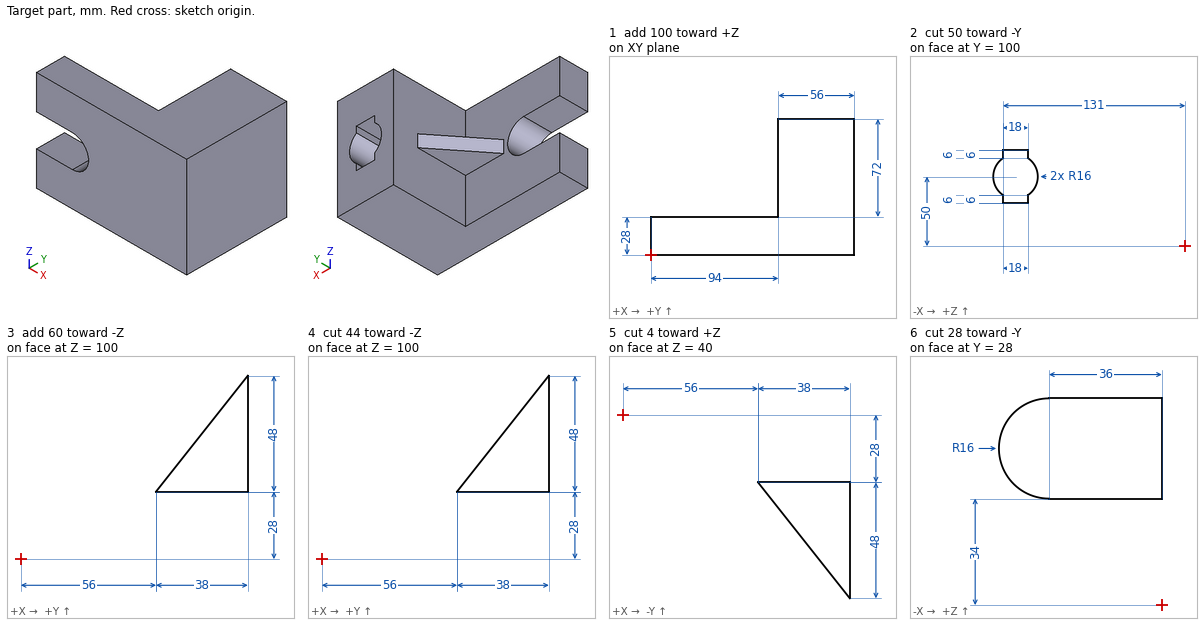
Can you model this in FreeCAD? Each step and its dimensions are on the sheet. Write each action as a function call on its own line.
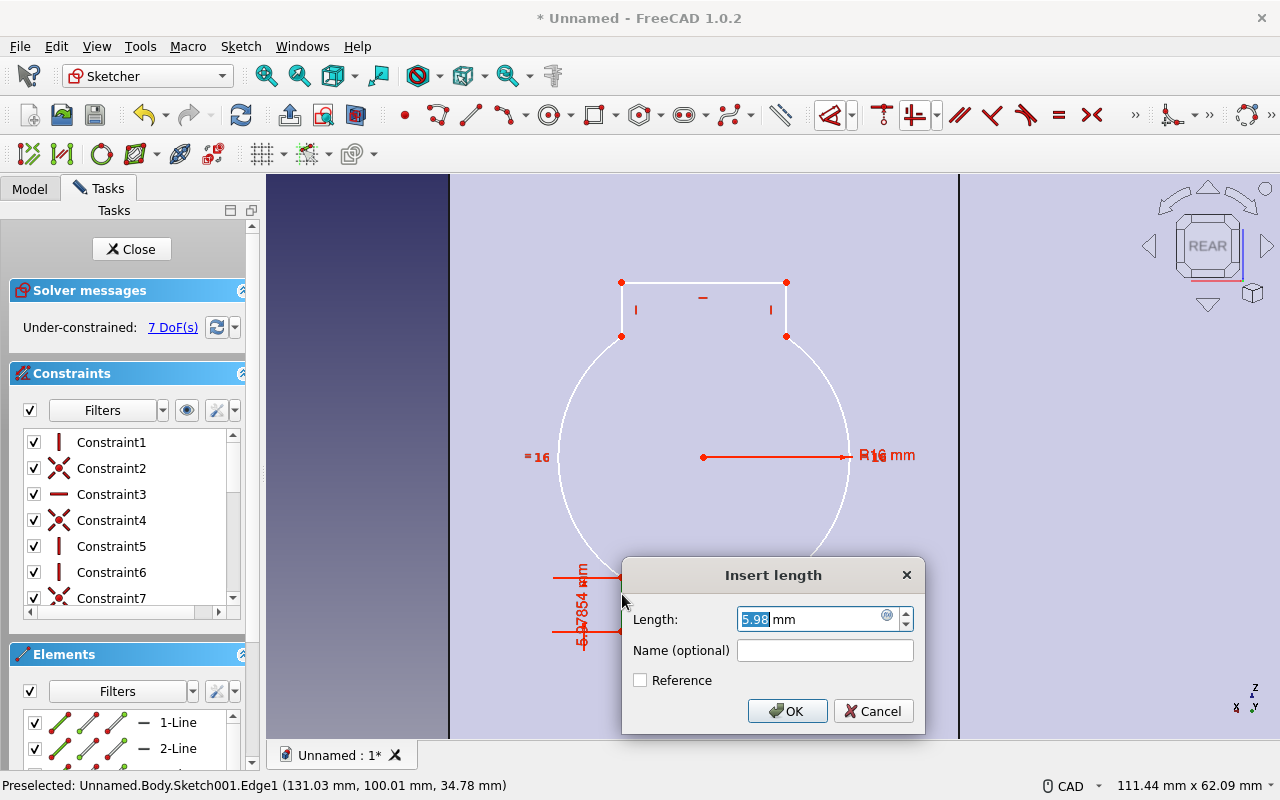
text(6)
key(Return)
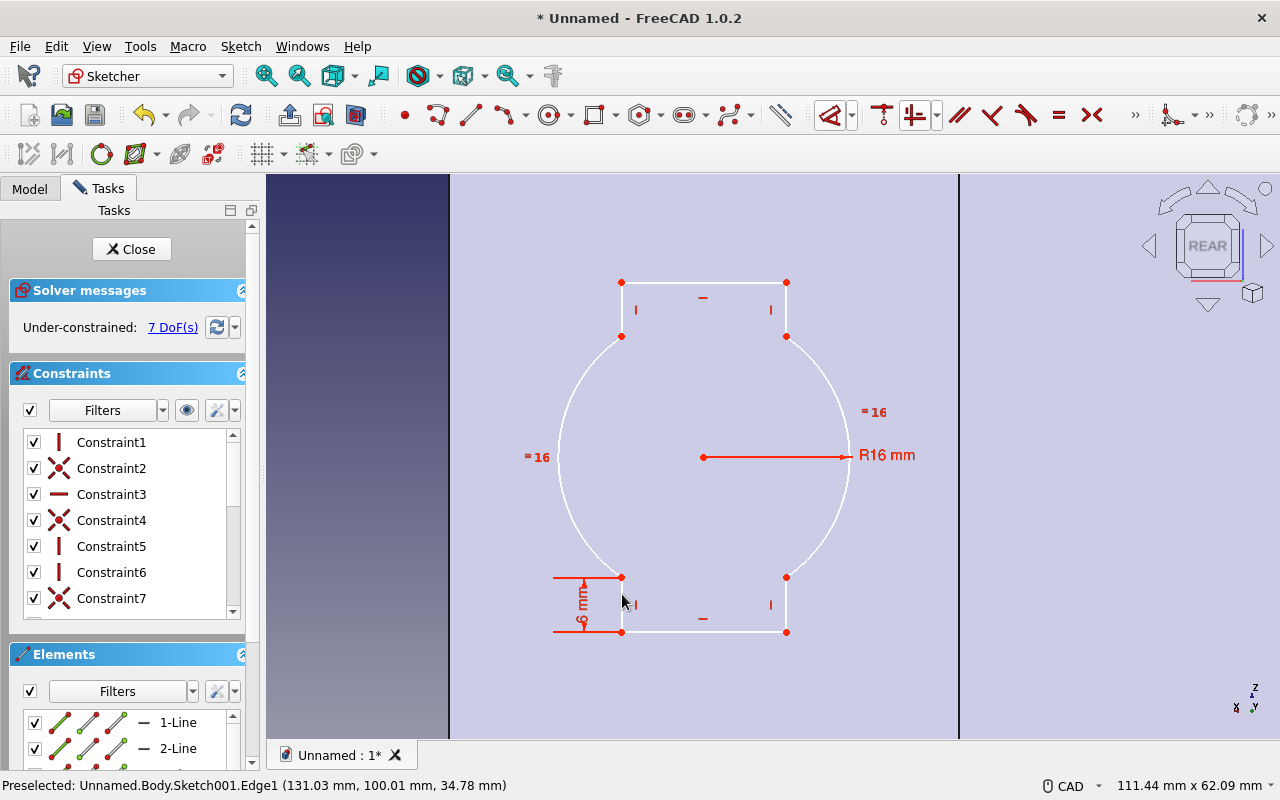
click(786, 616)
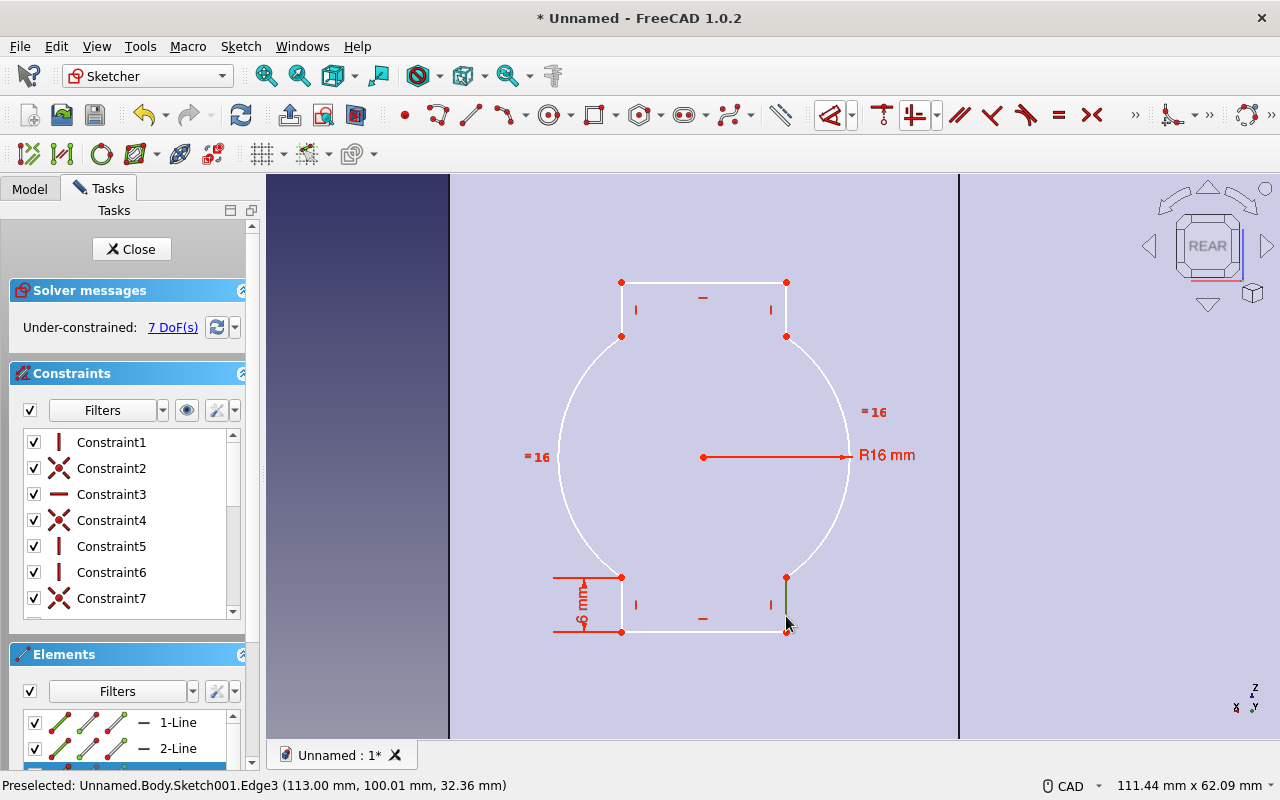
click(852, 116)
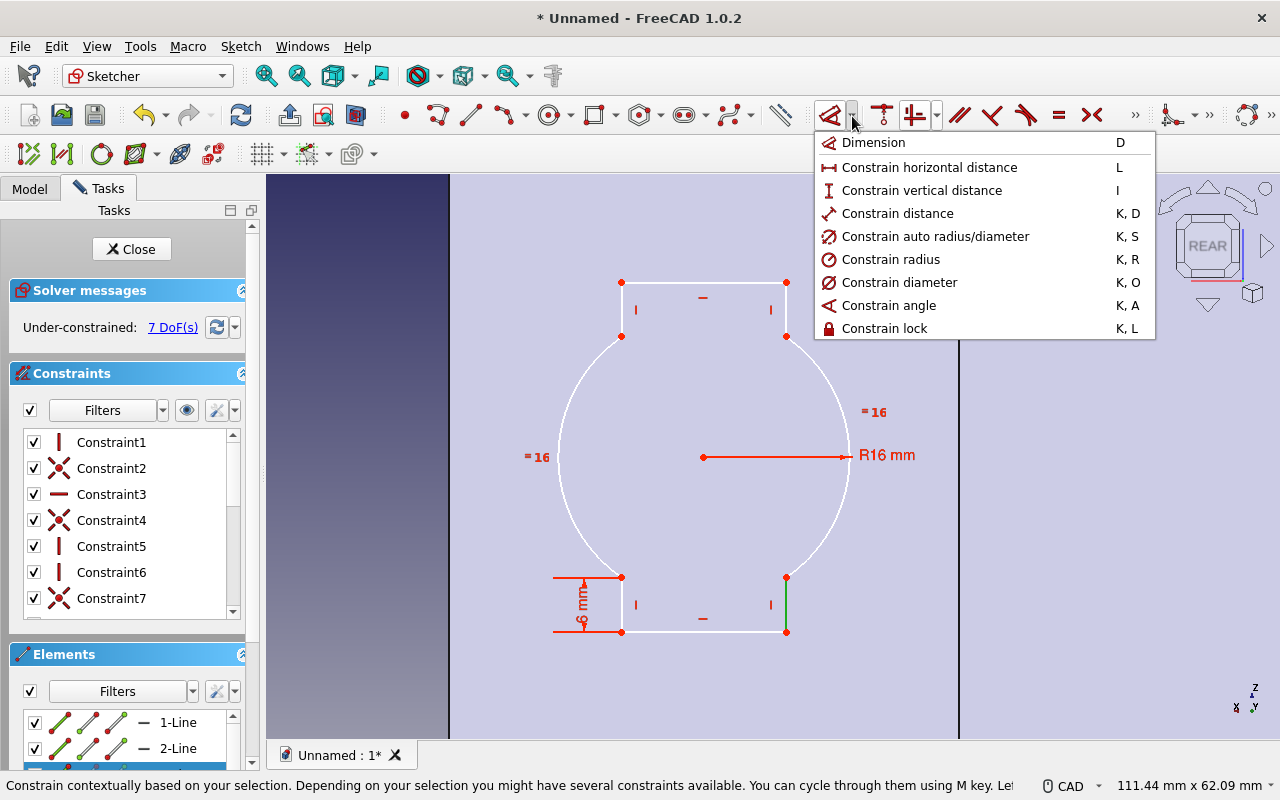
click(985, 190)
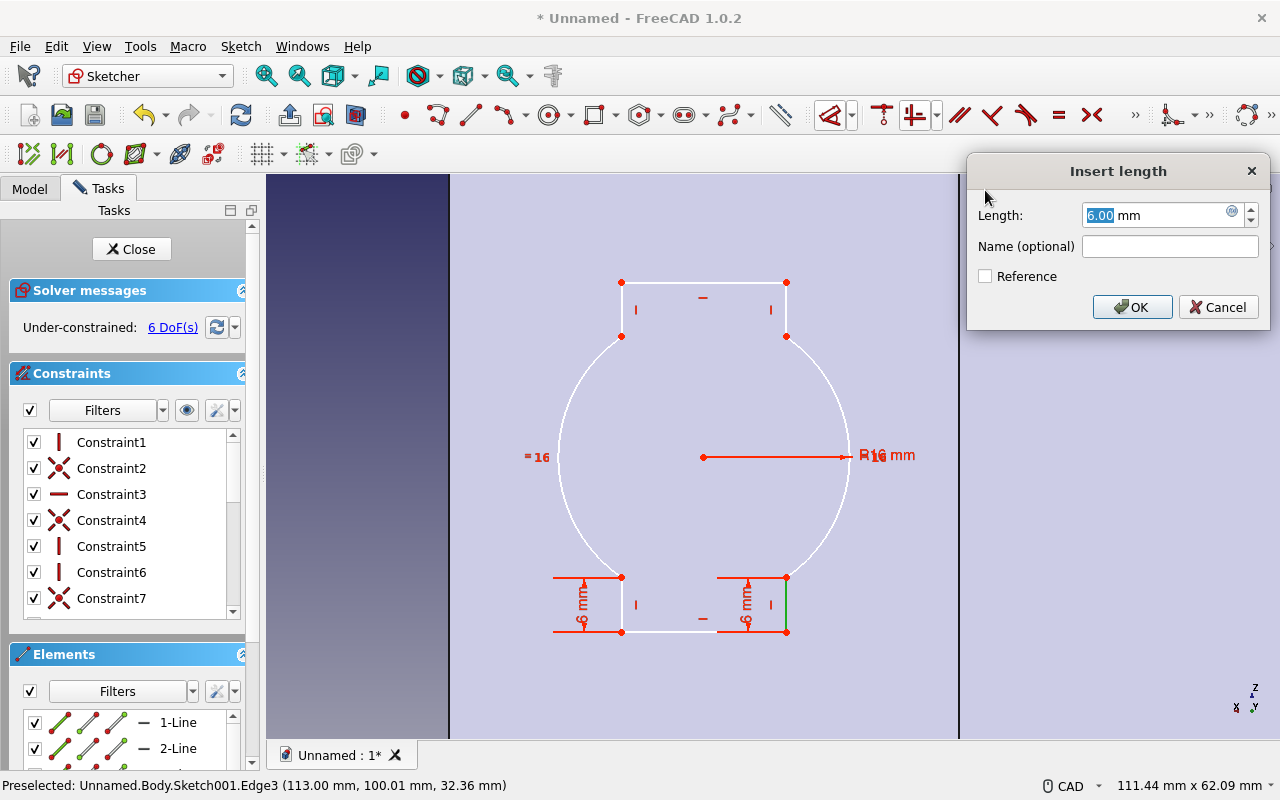
text(6)
key(Return)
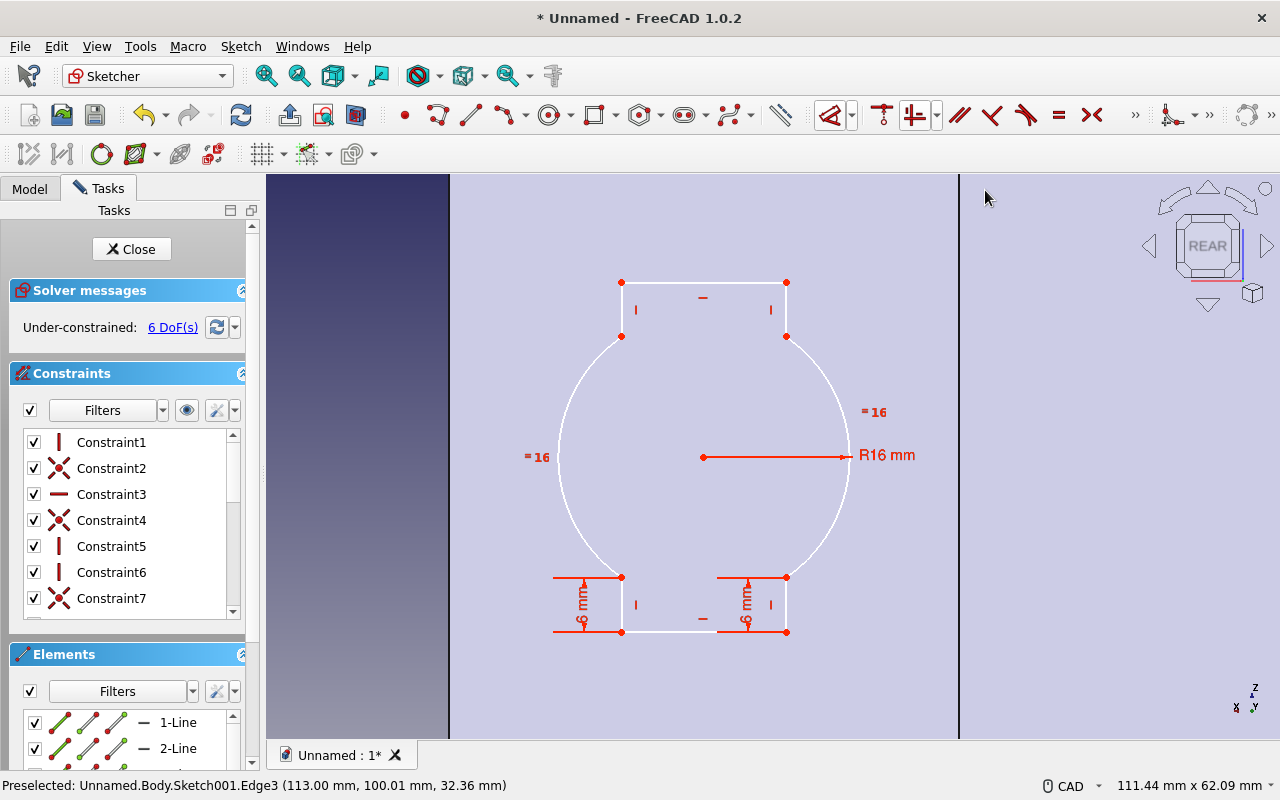
click(786, 321)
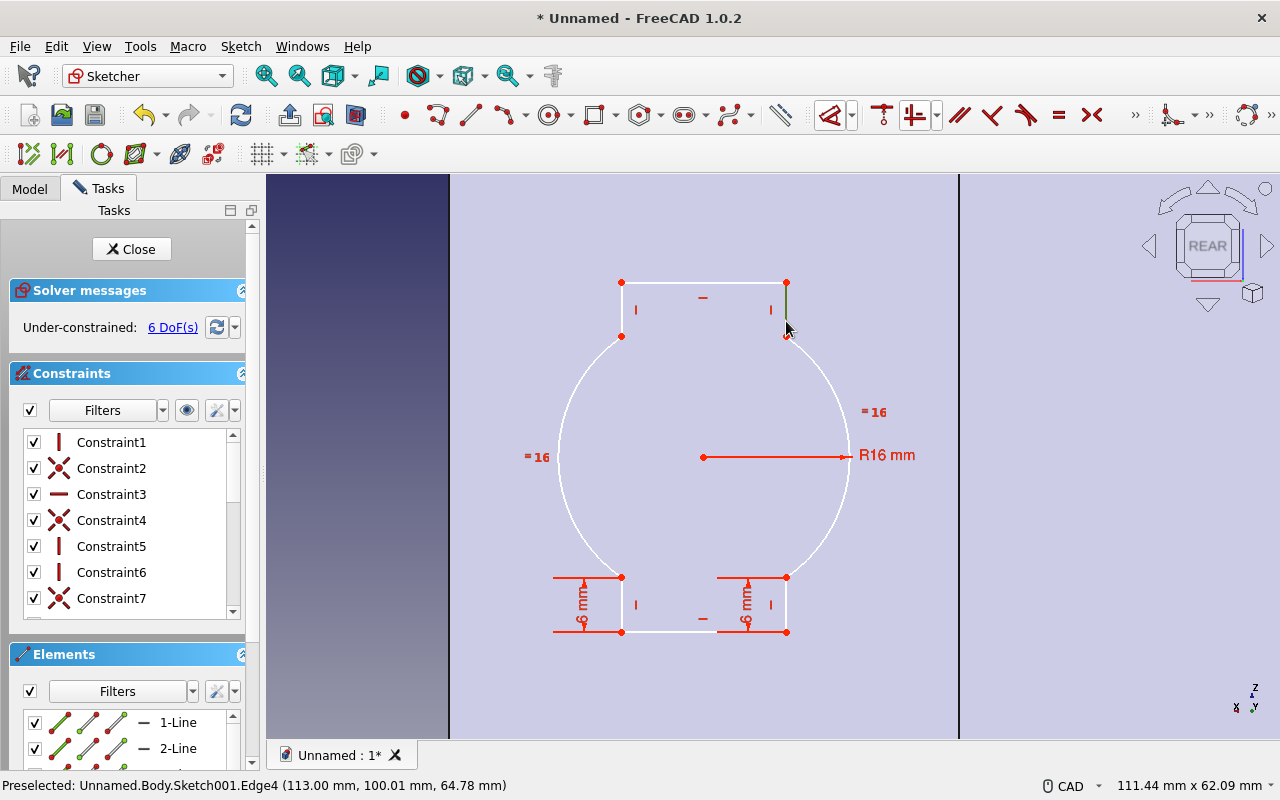
click(852, 116)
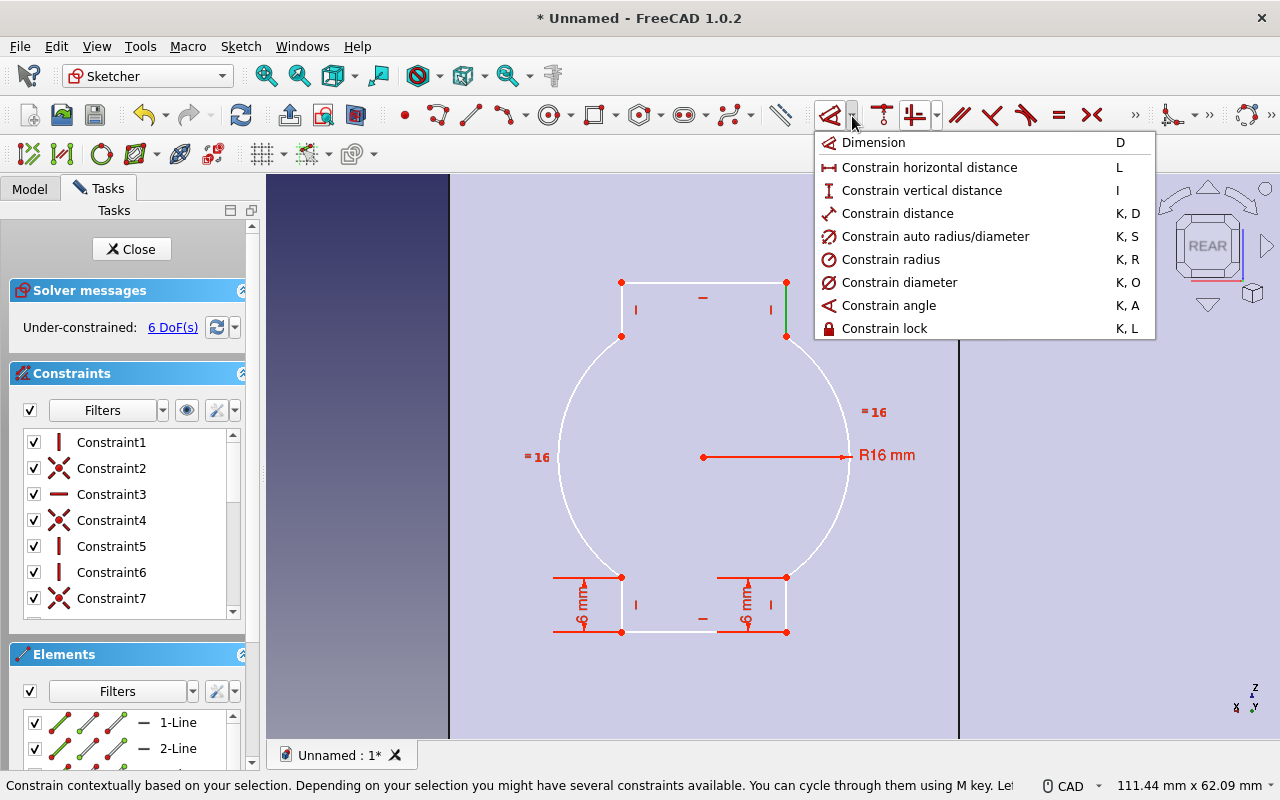
click(985, 190)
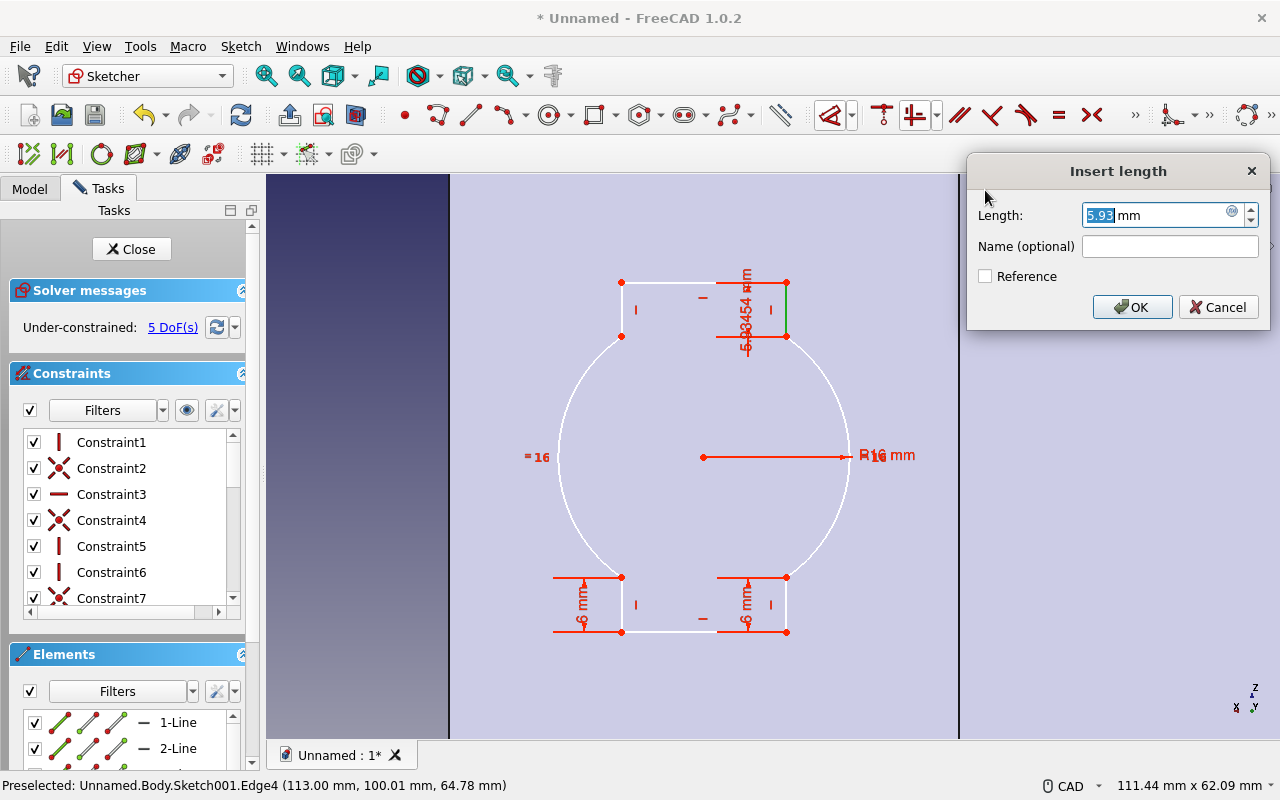
text(6)
key(Return)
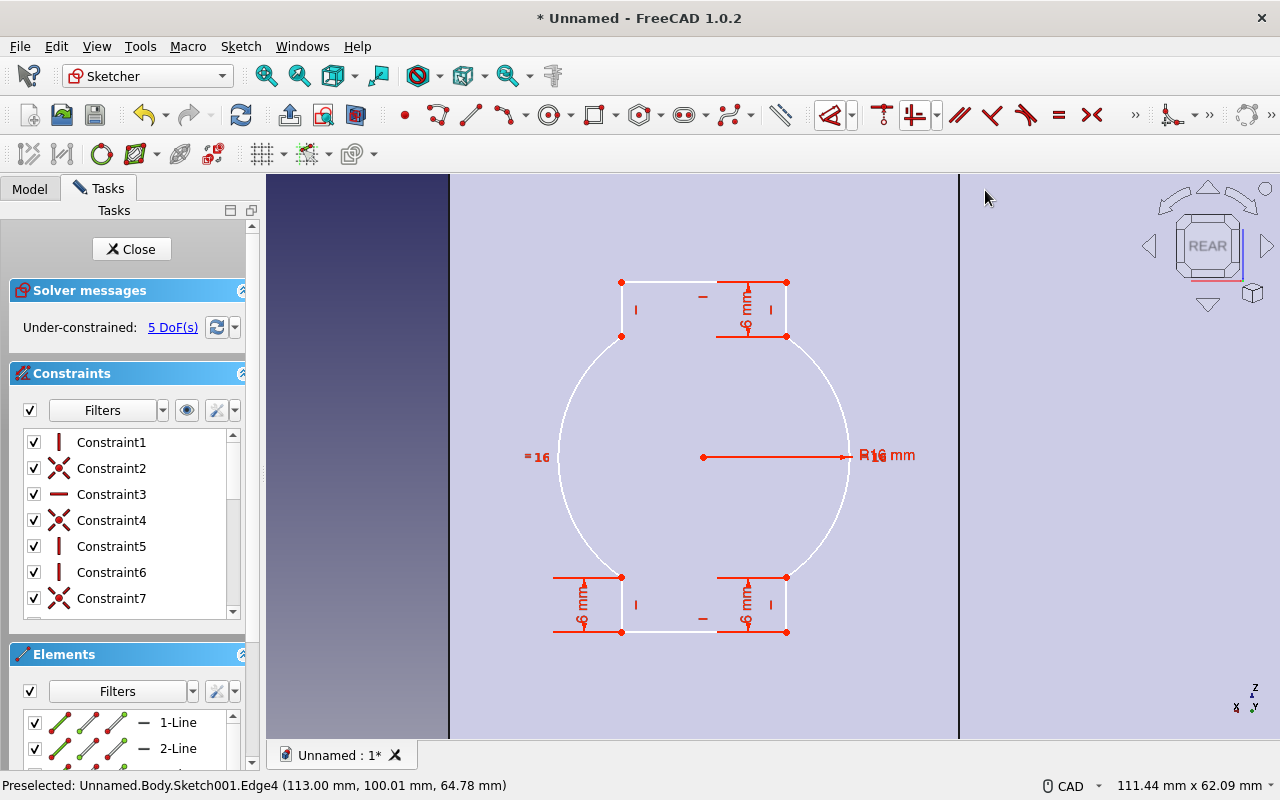
click(622, 299)